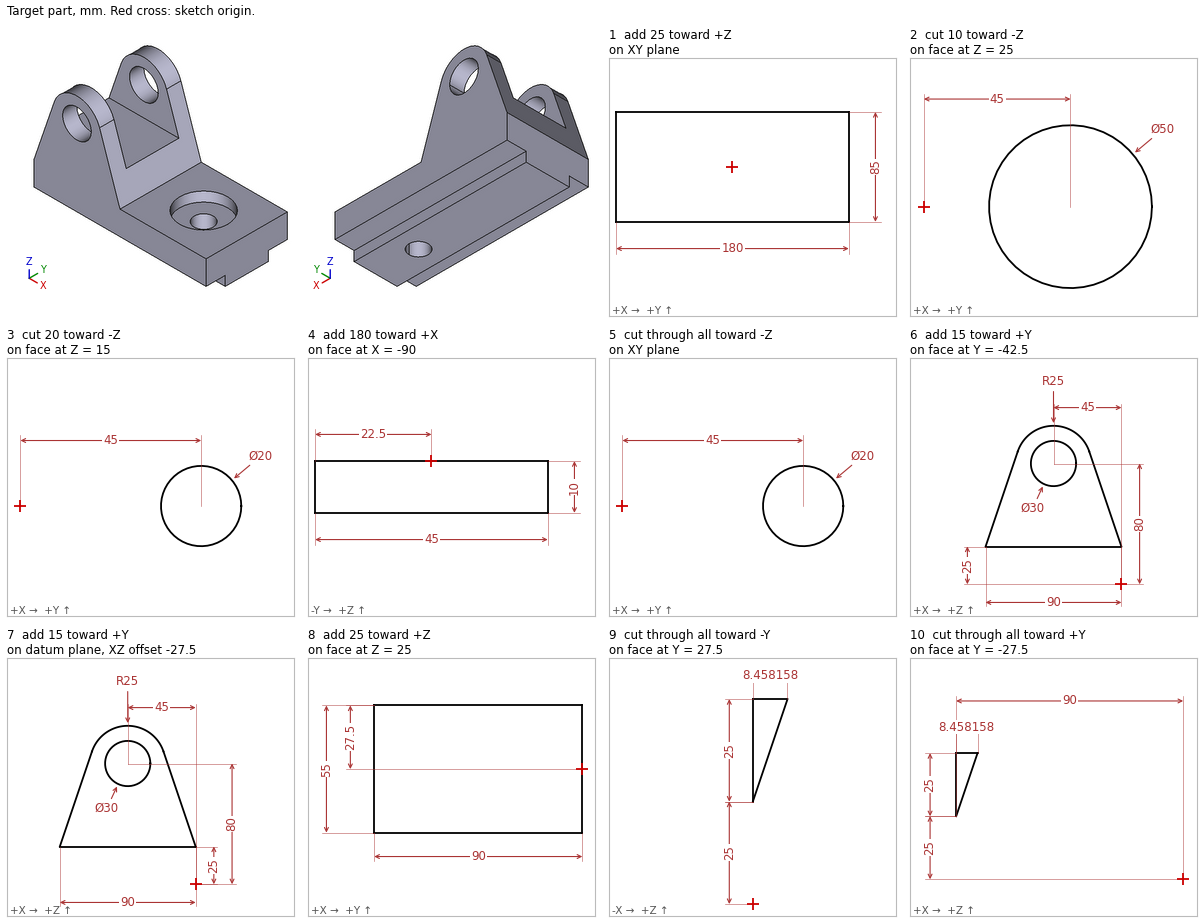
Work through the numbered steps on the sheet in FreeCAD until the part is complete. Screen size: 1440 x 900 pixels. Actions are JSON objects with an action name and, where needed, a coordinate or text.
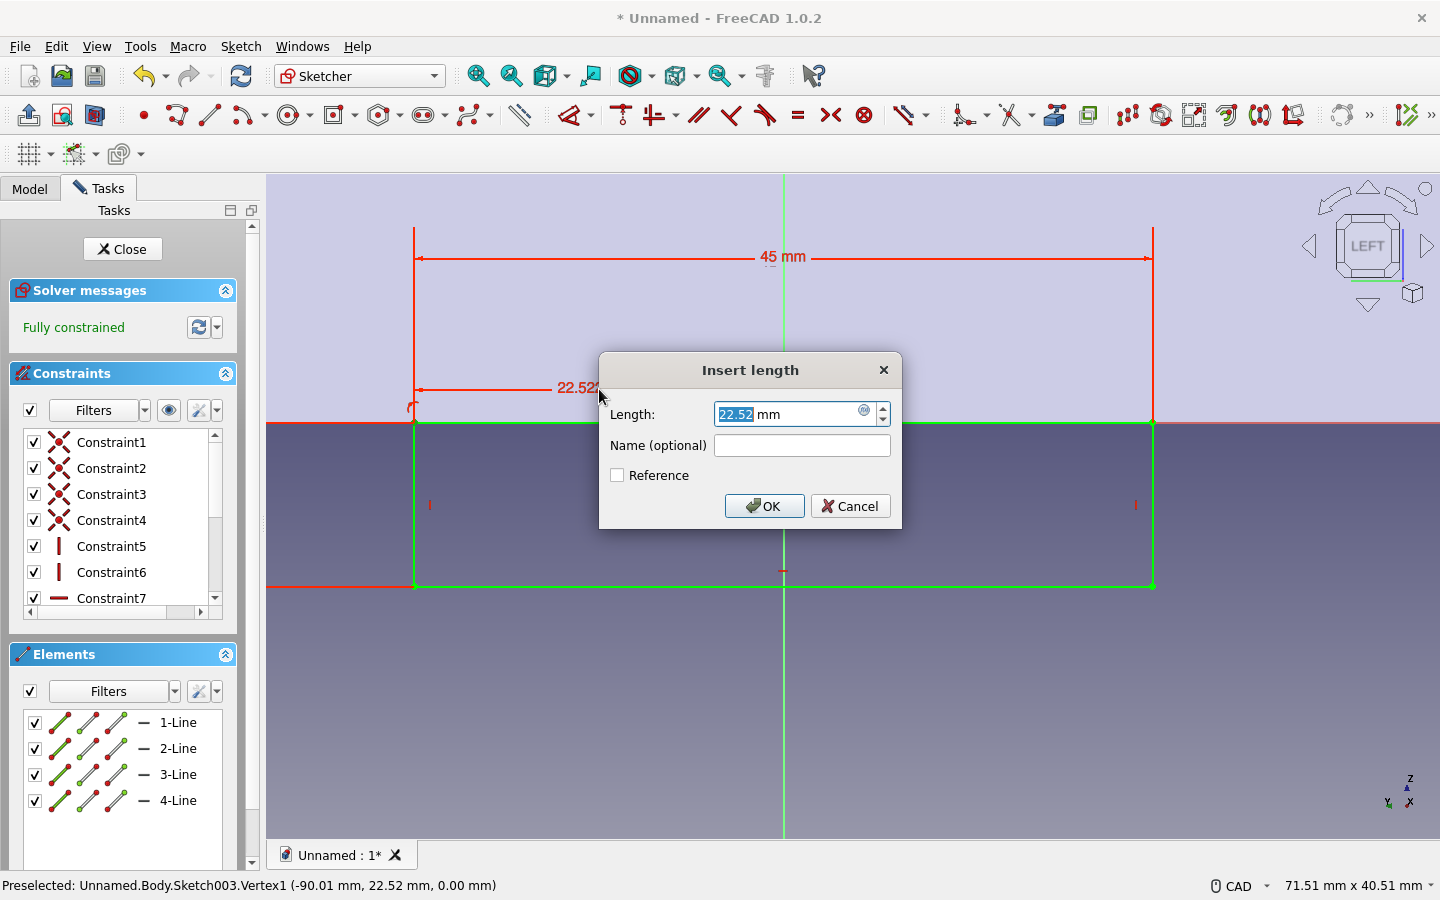
{"action": "type", "text": "22.5"}
{"action": "key", "text": "Return"}
{"action": "key", "text": "Escape"}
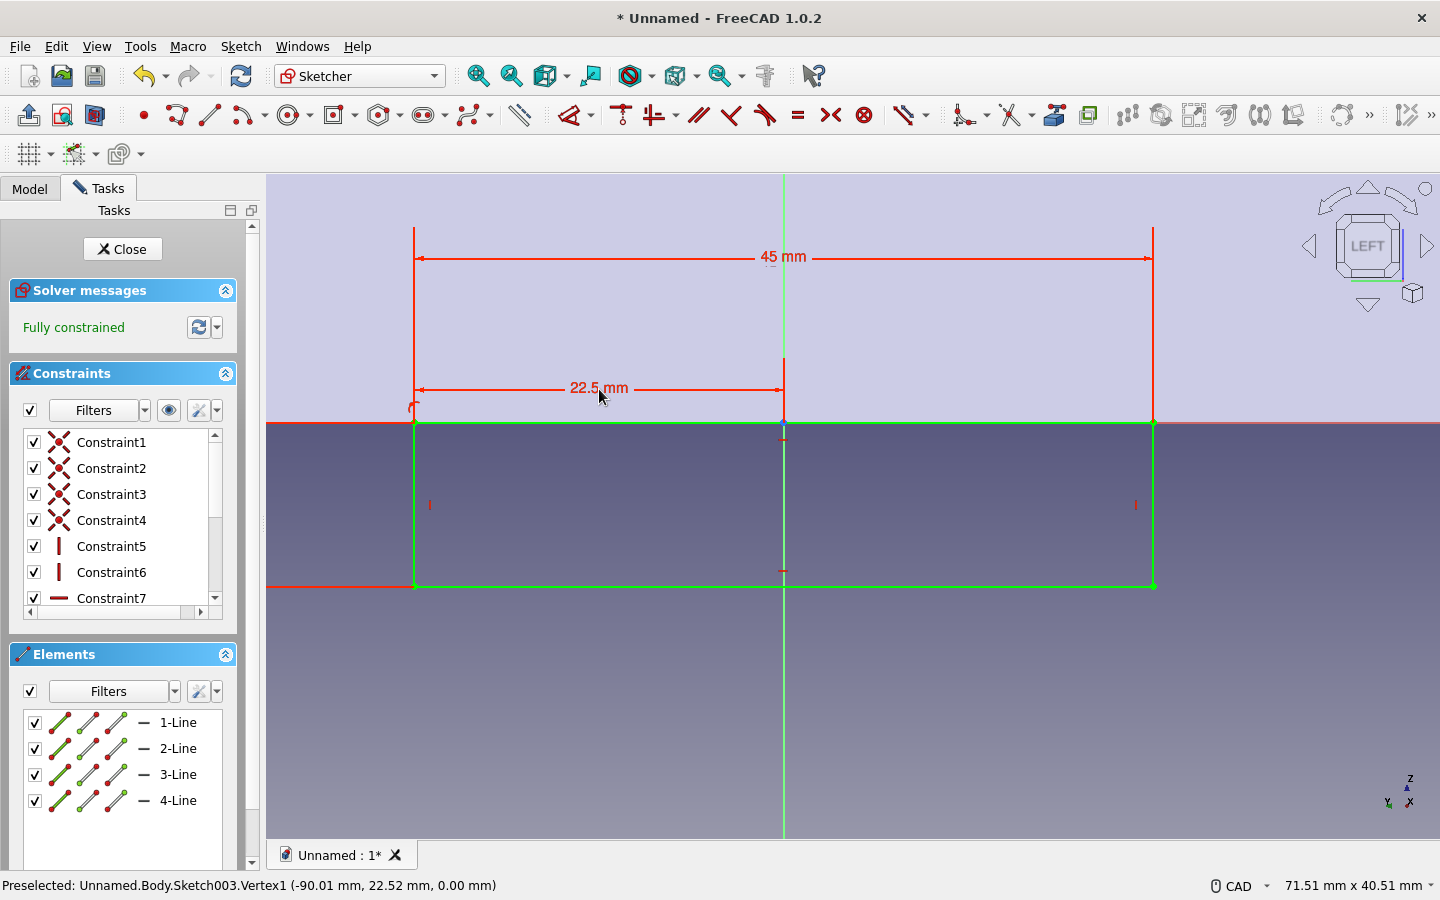
{"action": "left_click", "coordinate": [123, 249]}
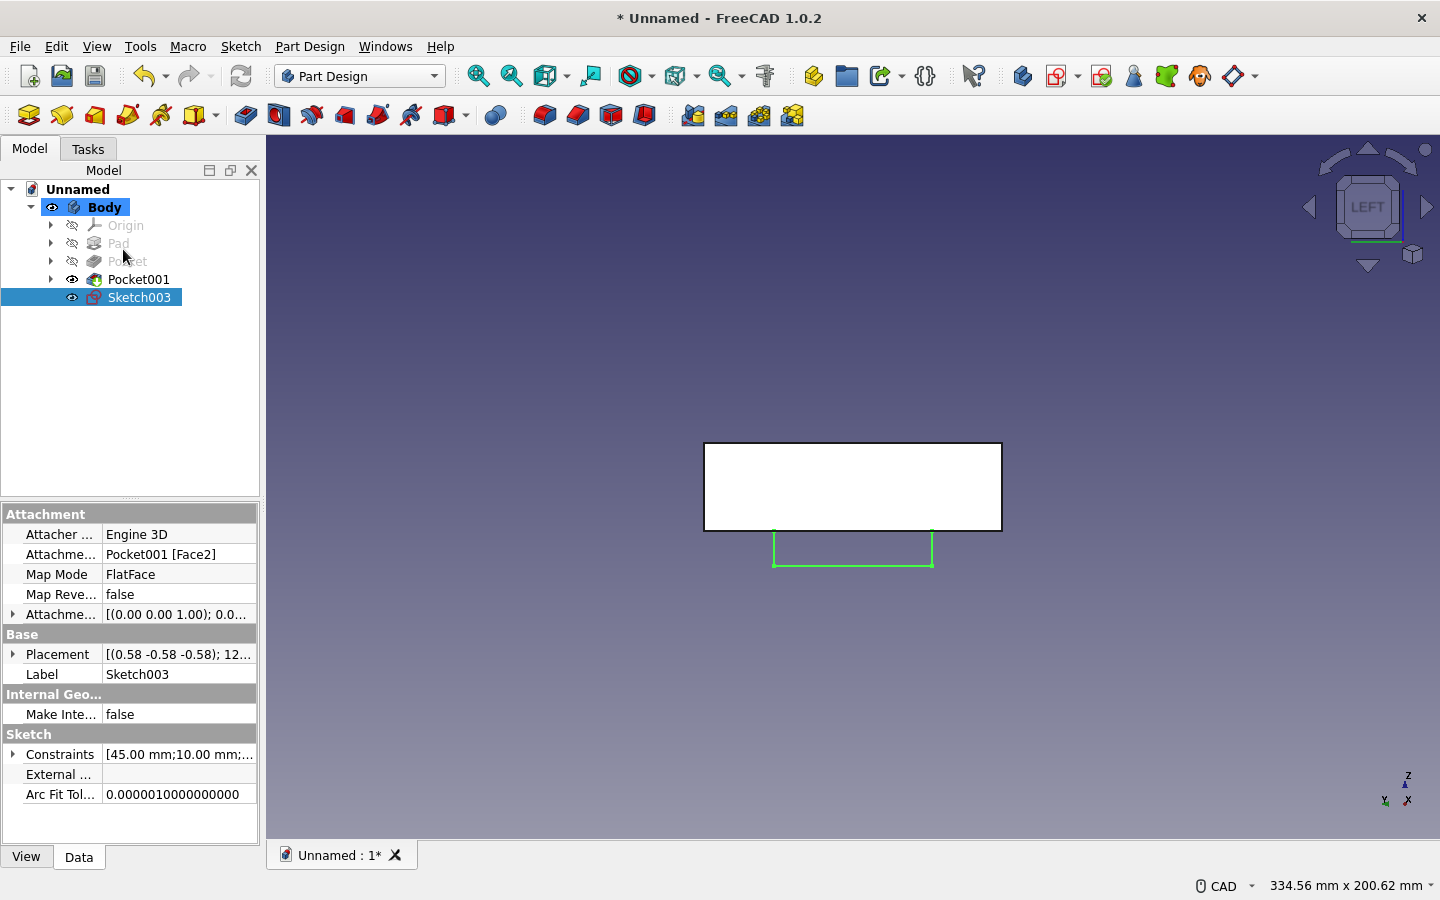
{"action": "left_click", "coordinate": [29, 116]}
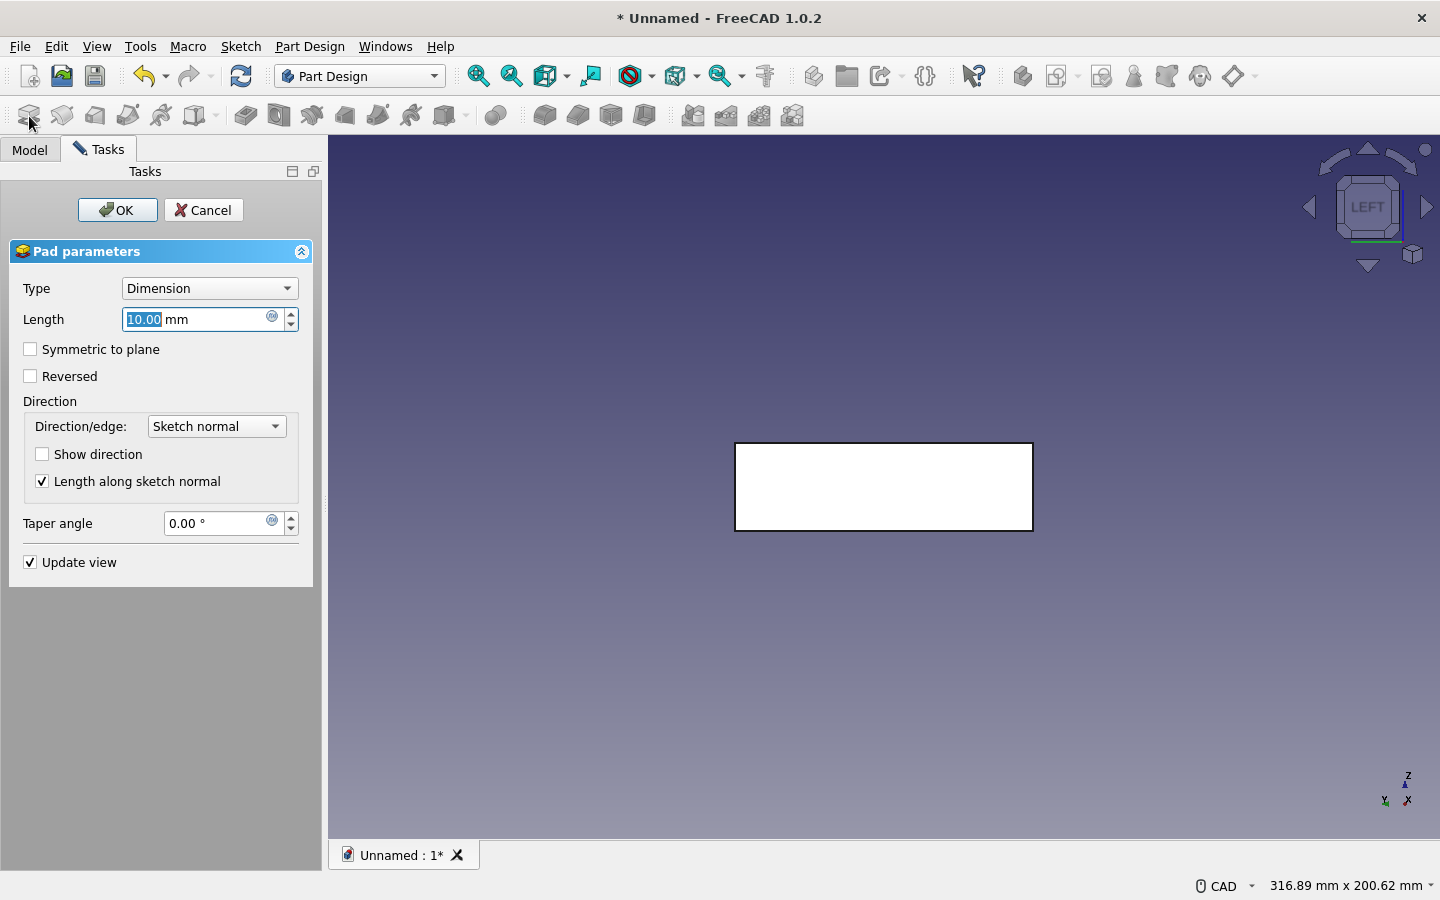
{"action": "type", "text": "180"}
{"action": "key", "text": "Tab"}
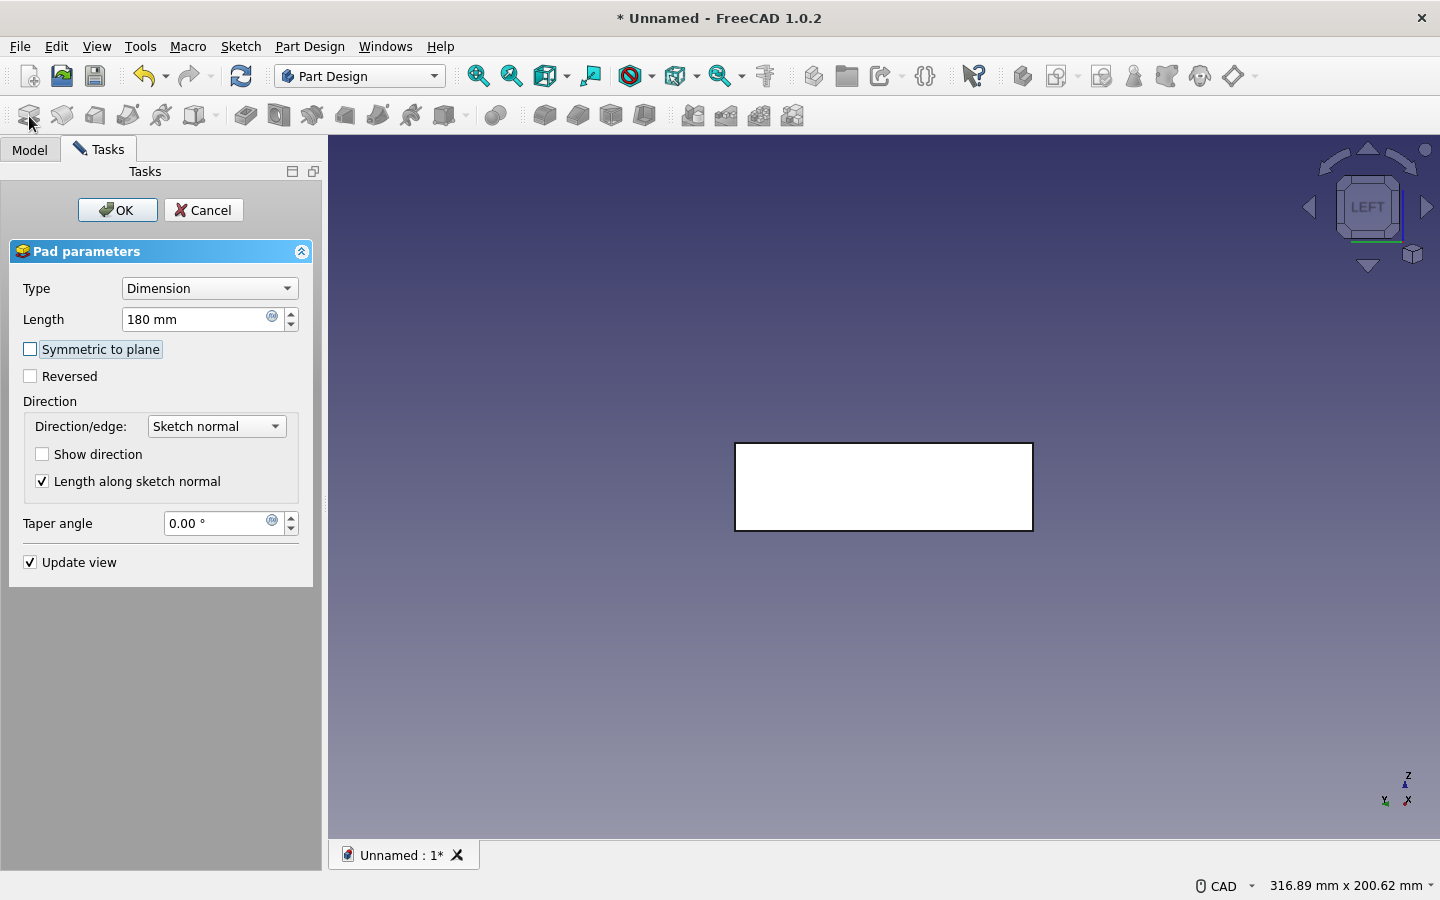
{"action": "left_click", "coordinate": [31, 376]}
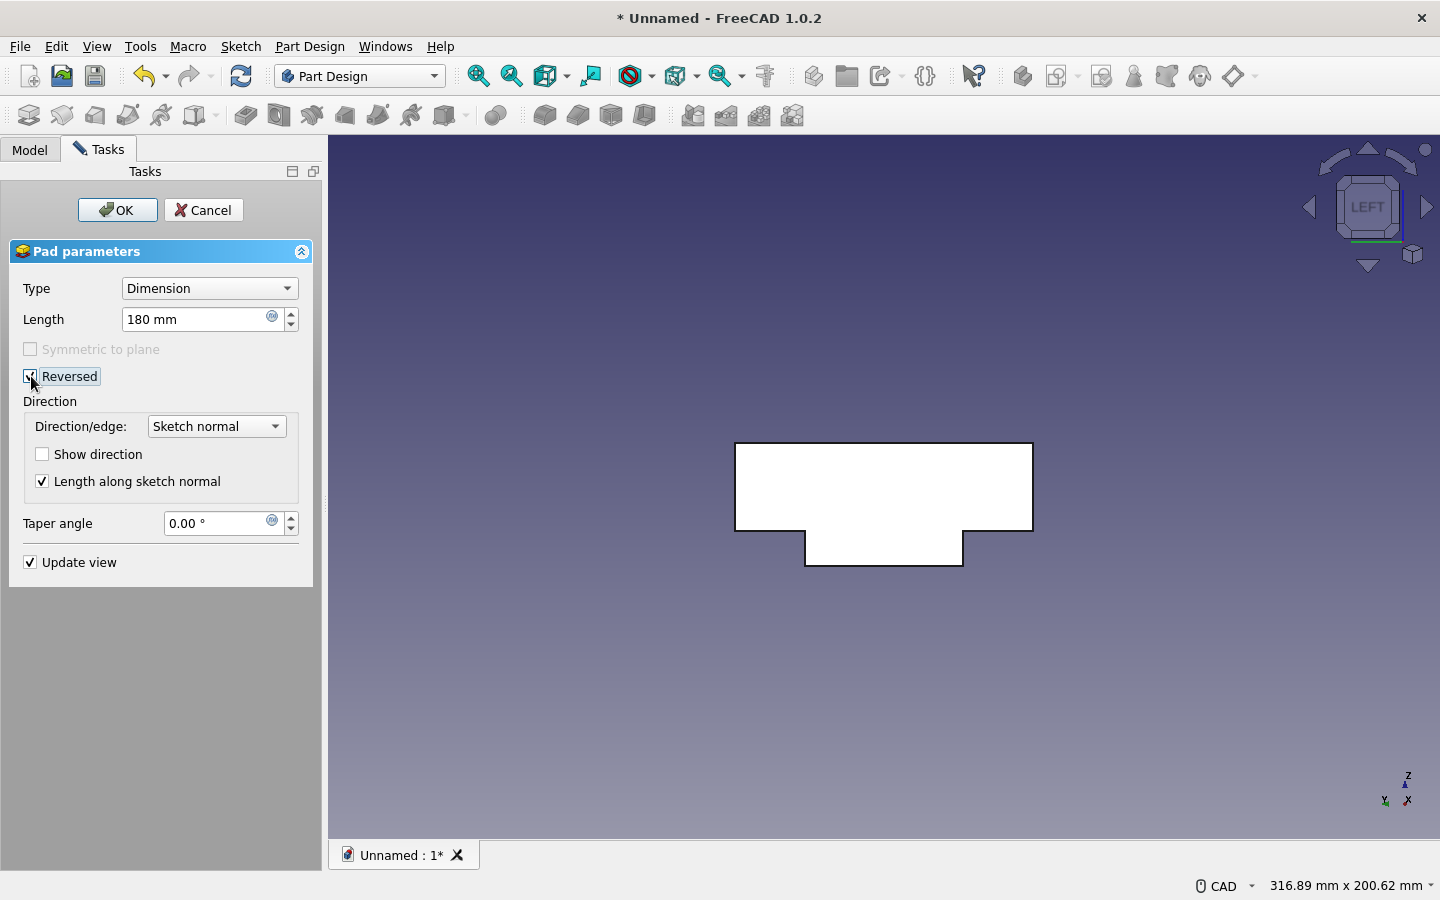
{"action": "left_click", "coordinate": [118, 210]}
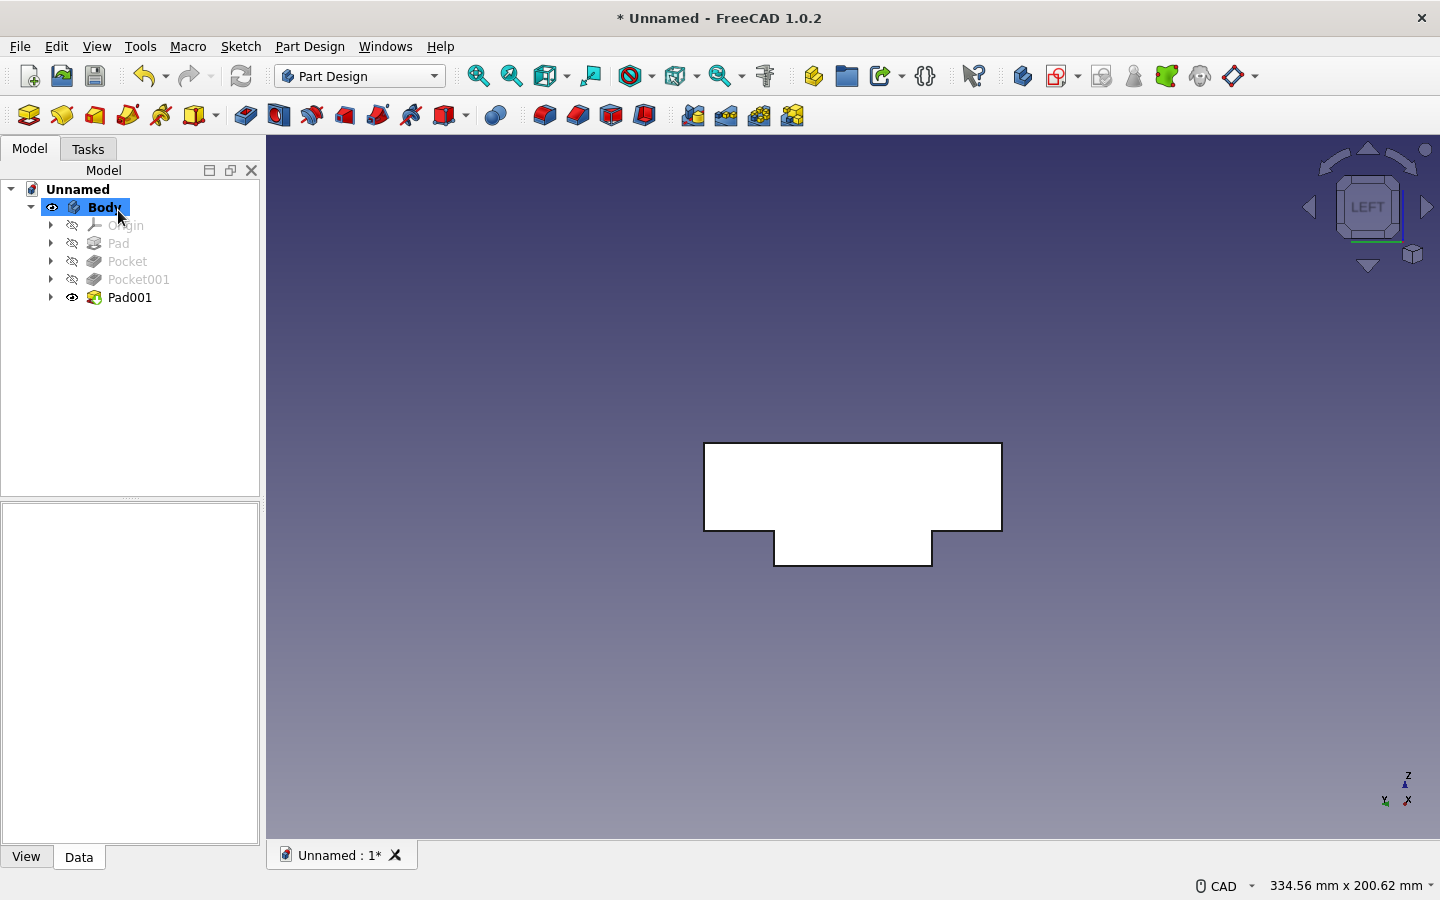
{"action": "left_click", "coordinate": [479, 76]}